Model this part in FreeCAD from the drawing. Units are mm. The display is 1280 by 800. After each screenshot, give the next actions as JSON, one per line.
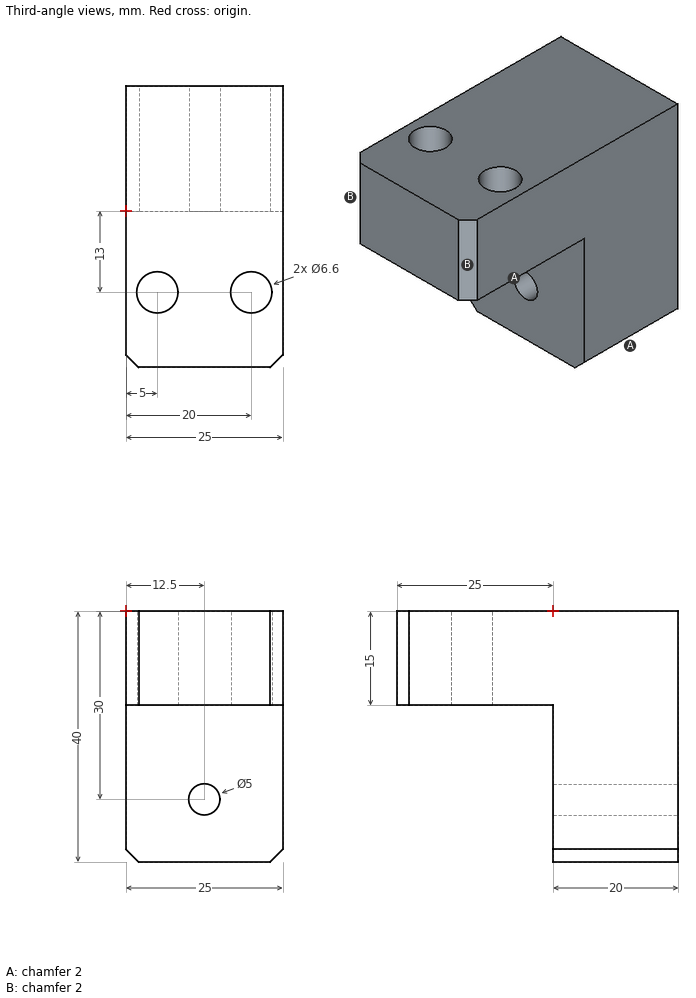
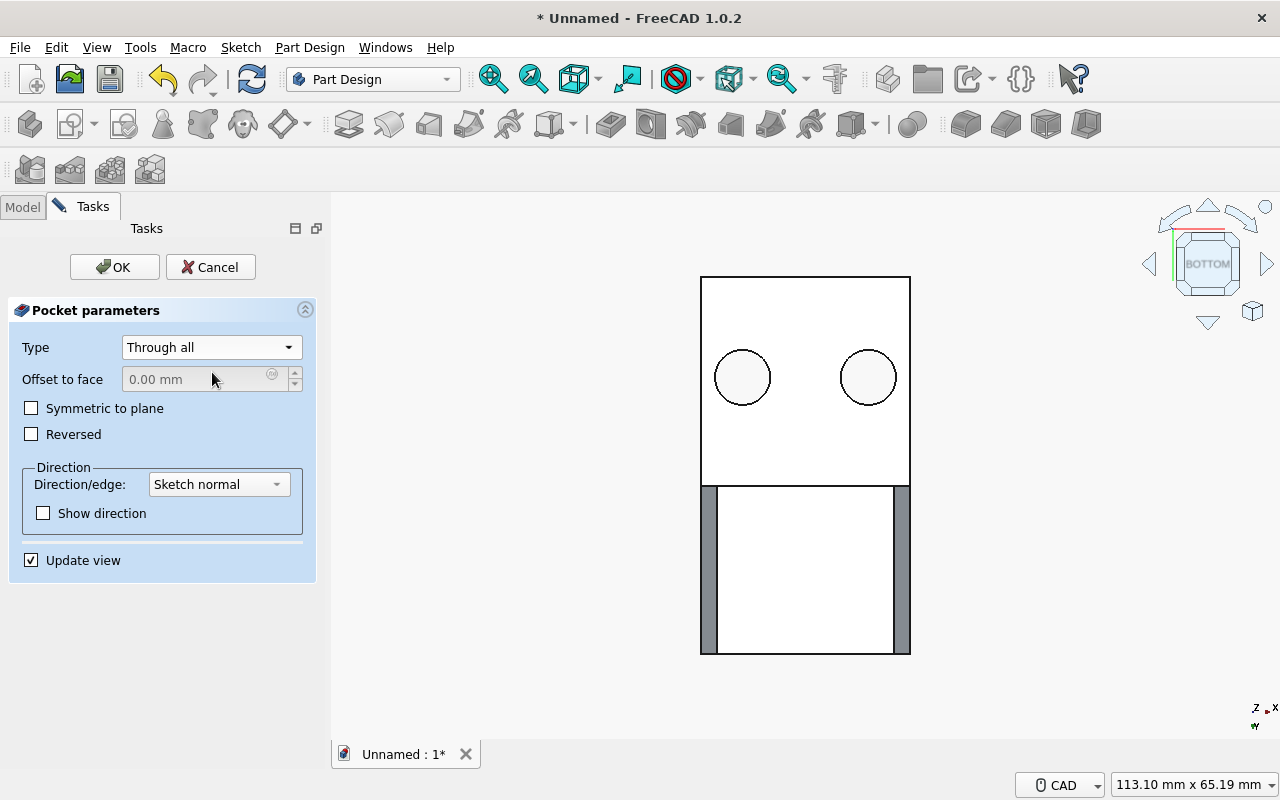
{"action": "left_click", "coordinate": [115, 267]}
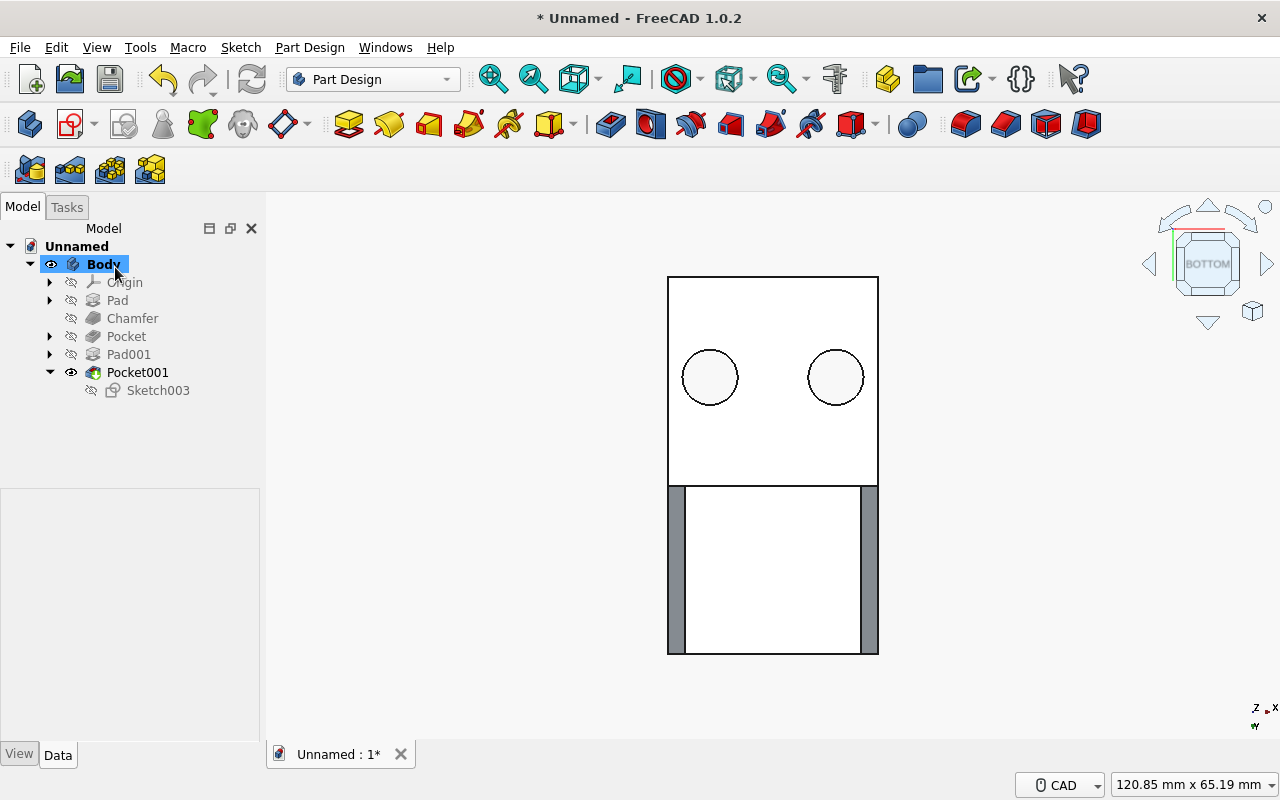
{"action": "key", "text": "0"}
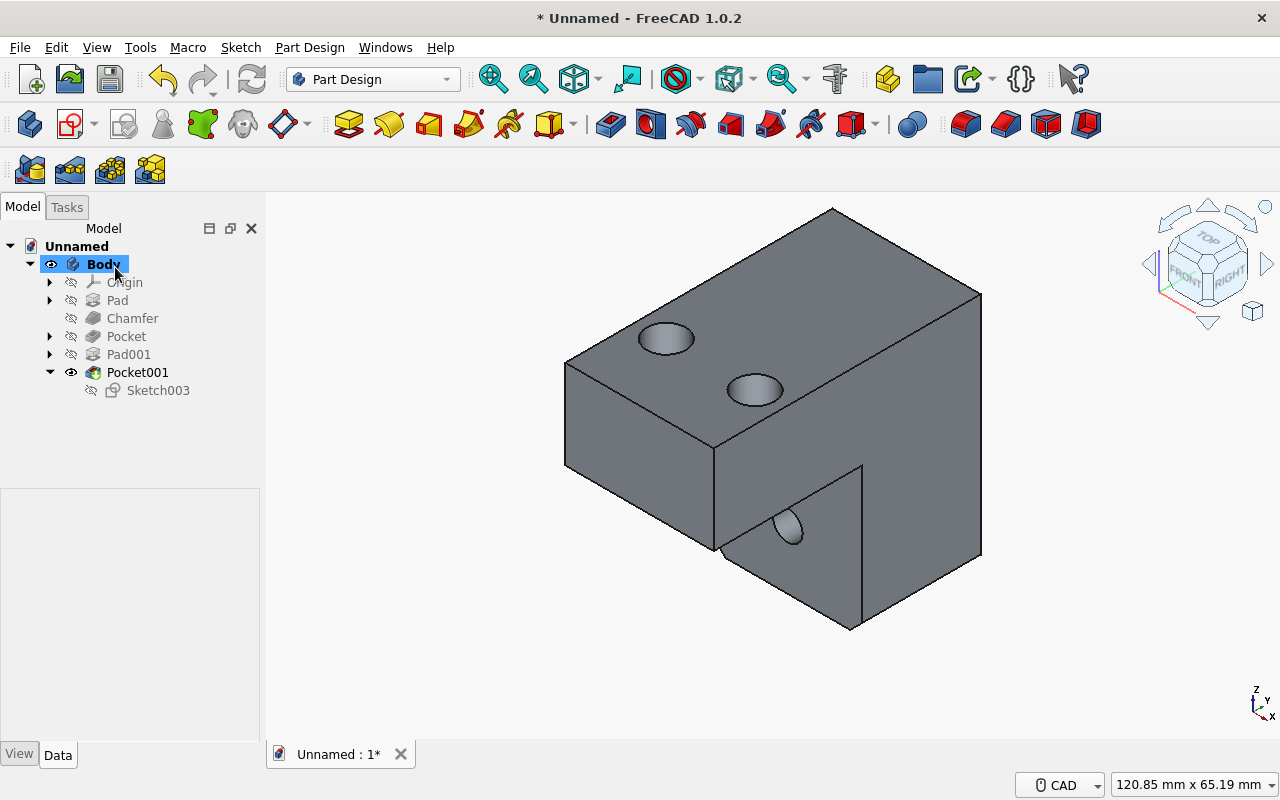
{"action": "left_click", "coordinate": [714, 499]}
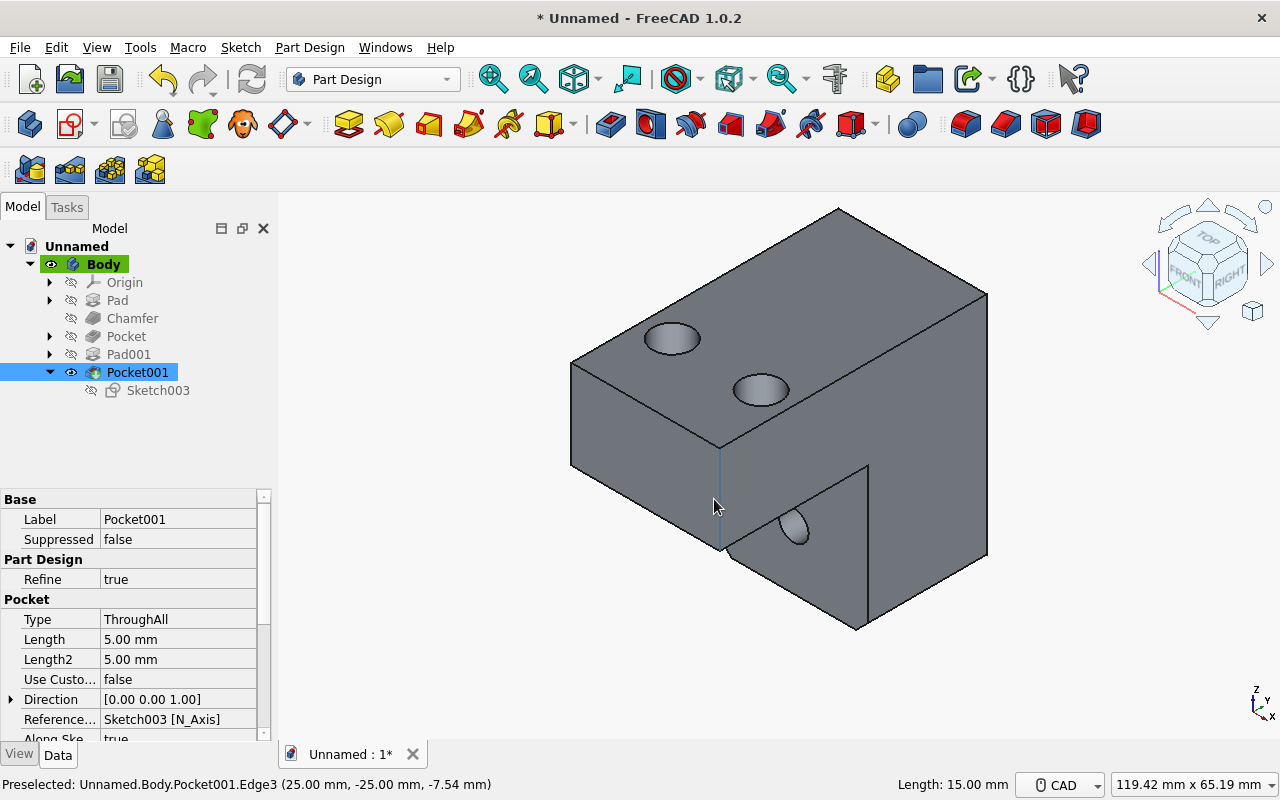
{"action": "key", "text": "2"}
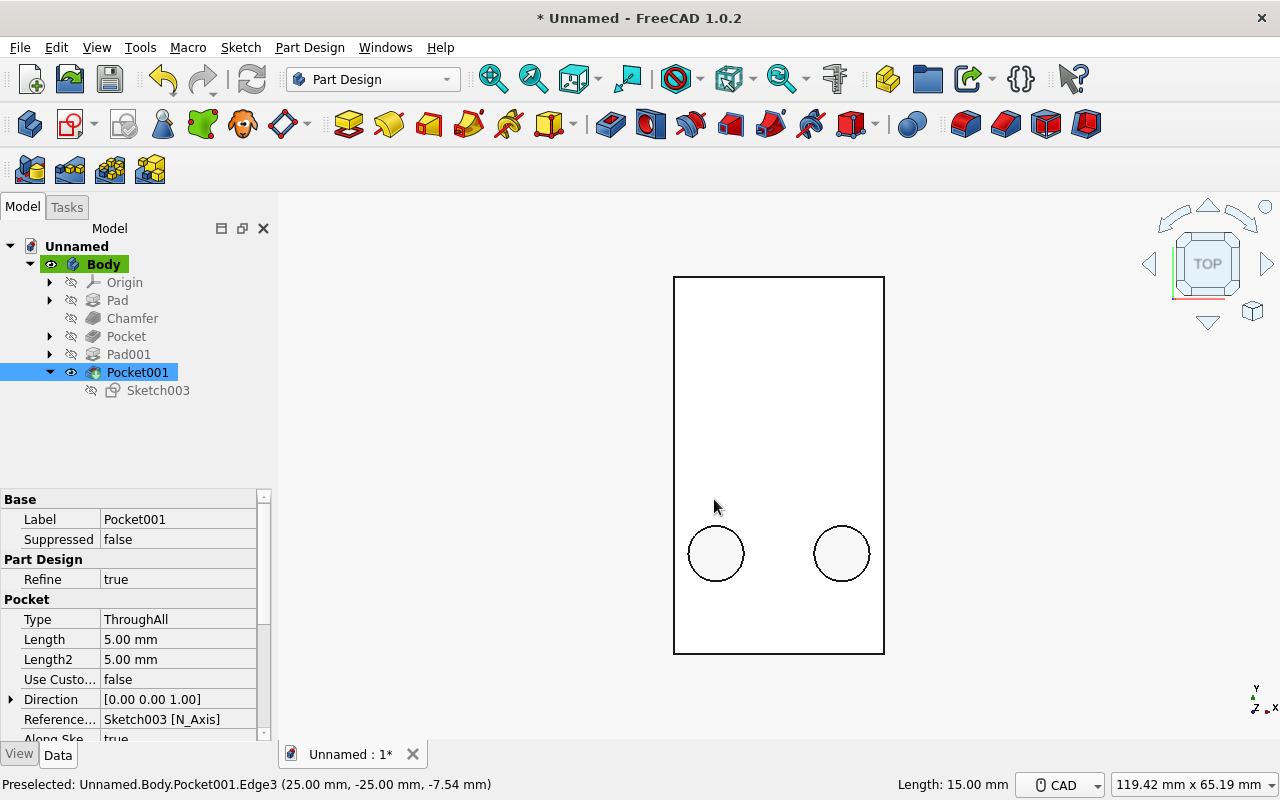
{"action": "key", "text": "1"}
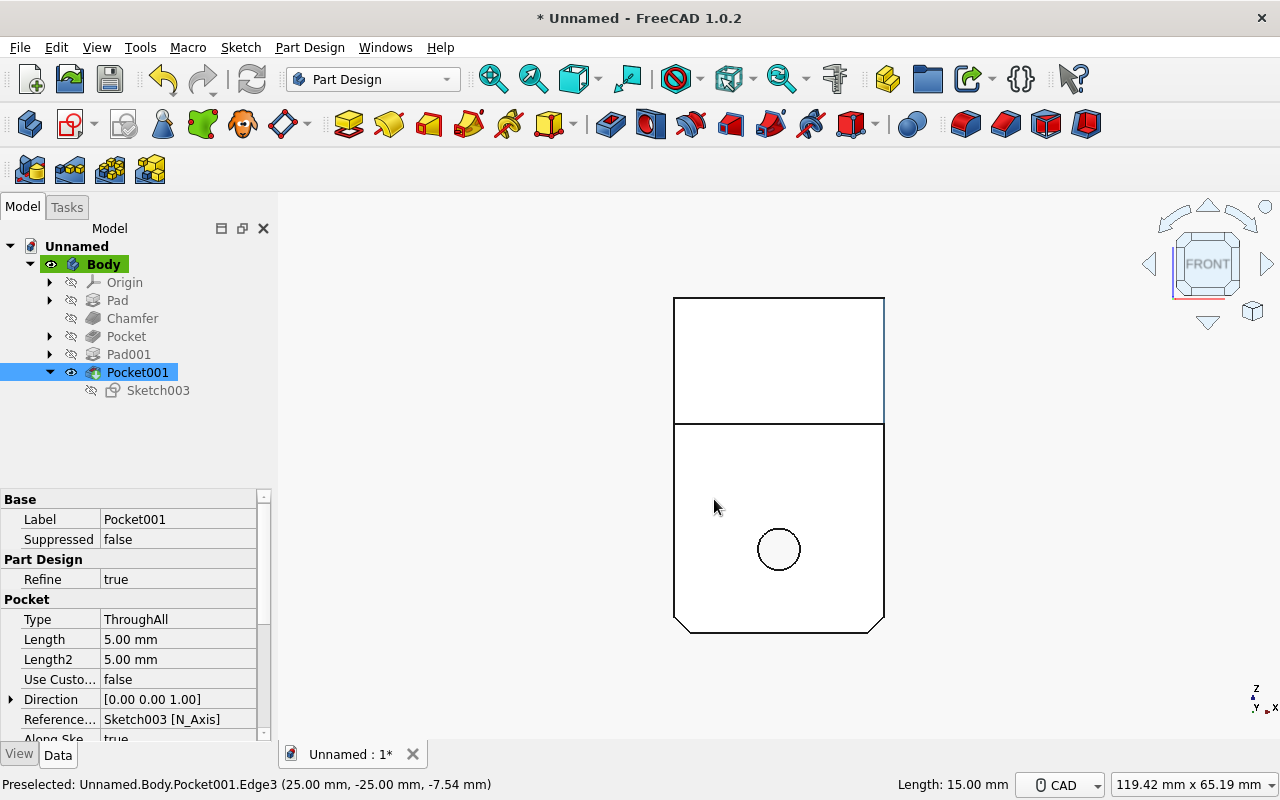
{"action": "left_click", "coordinate": [674, 360], "text": "ctrl"}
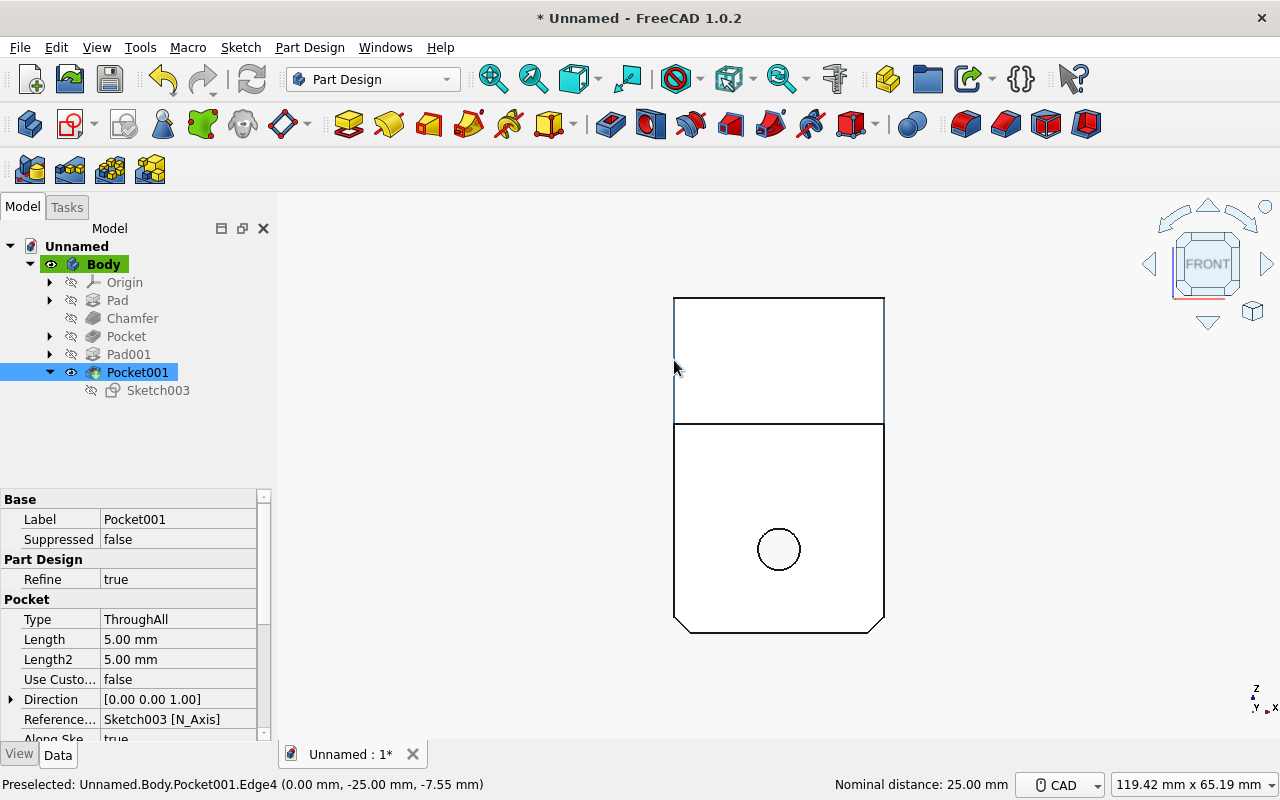
{"action": "left_click", "coordinate": [1006, 124]}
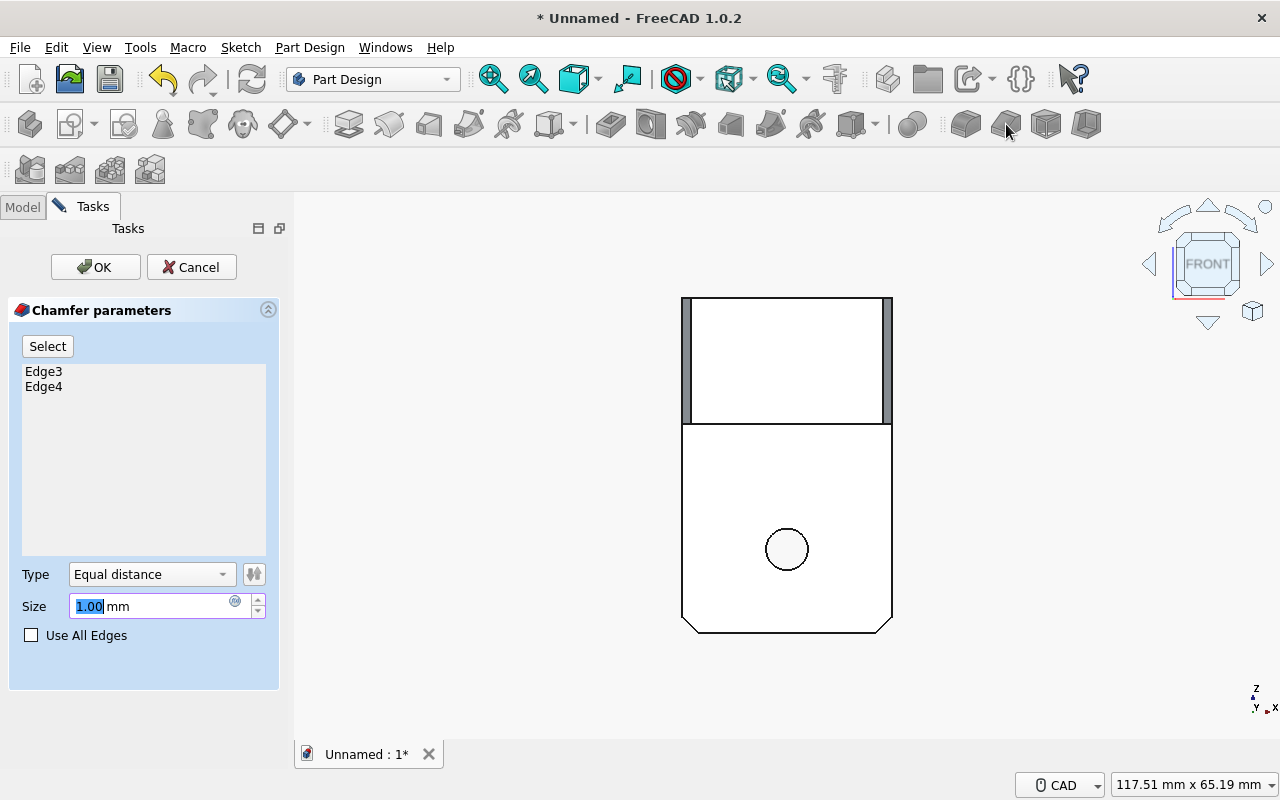
{"action": "type", "text": "2"}
{"action": "key", "text": "Tab"}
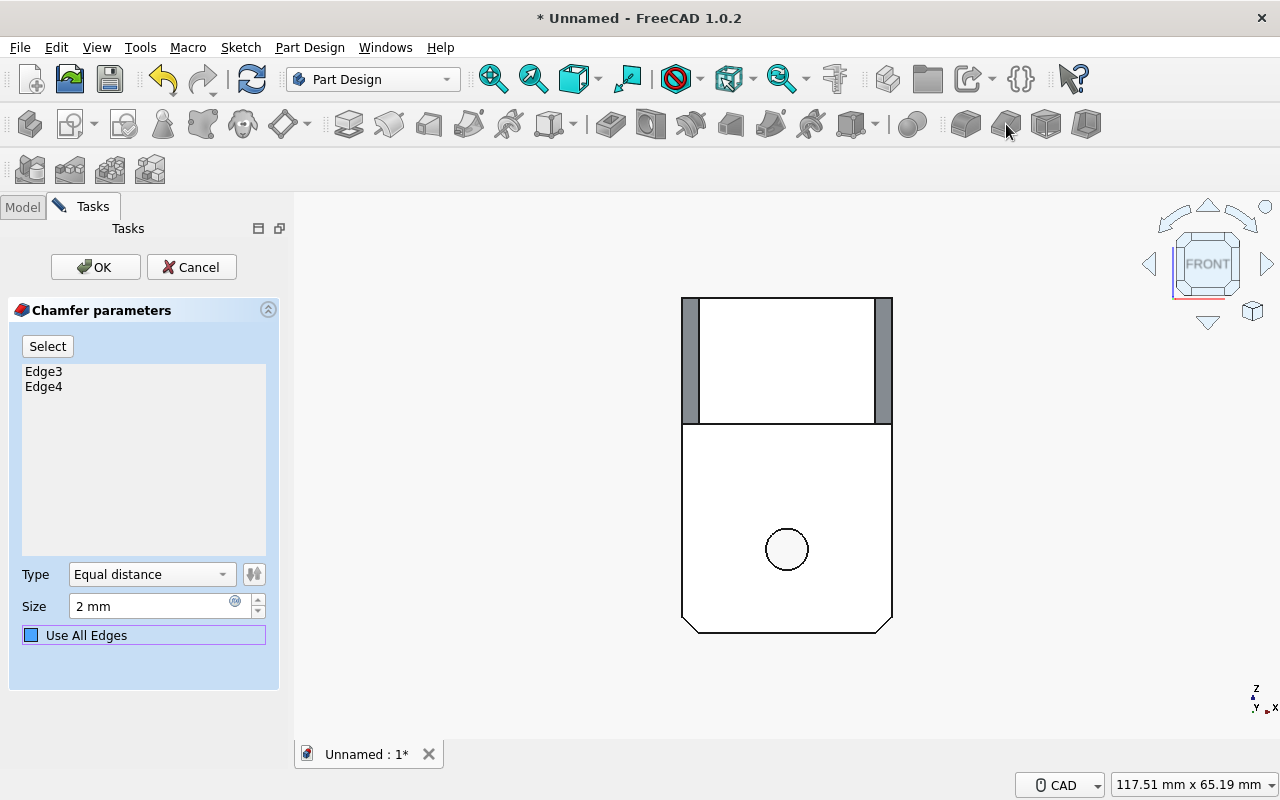
{"action": "left_click", "coordinate": [96, 267]}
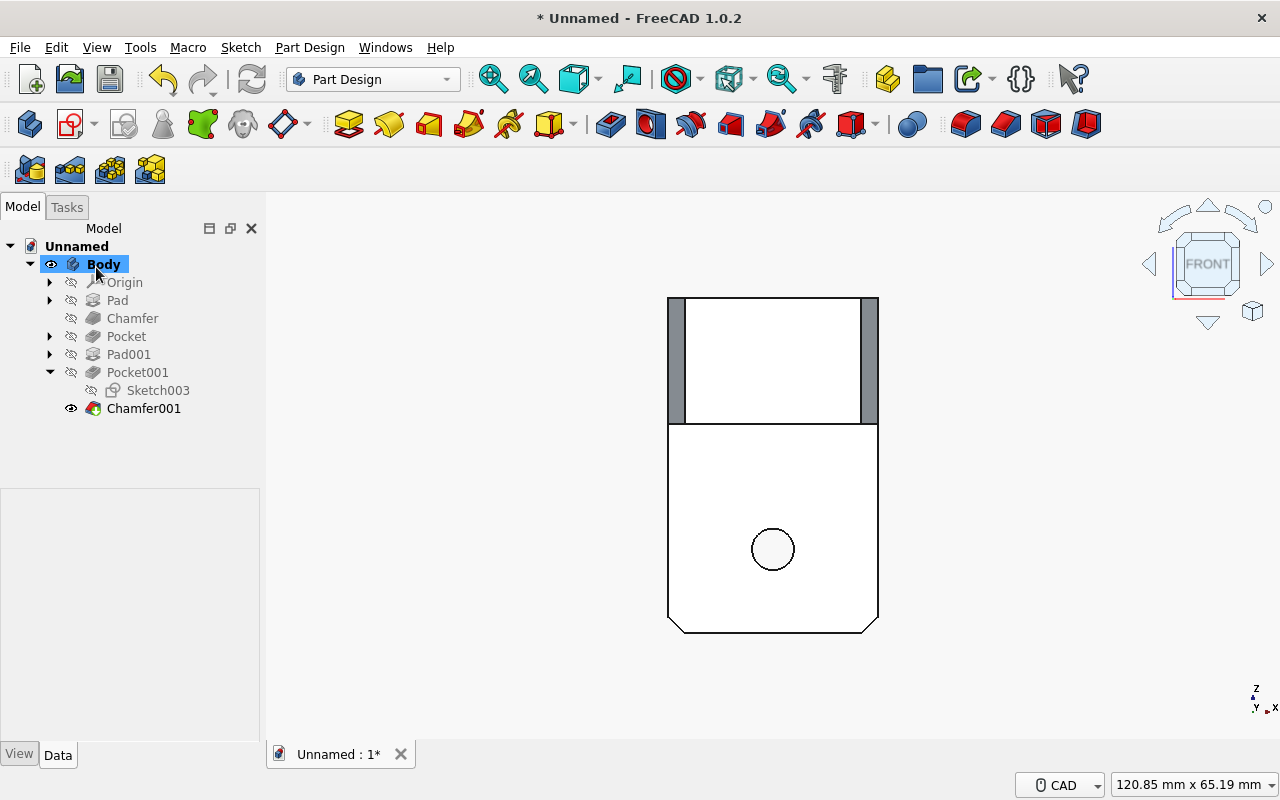
{"action": "key", "text": "0"}